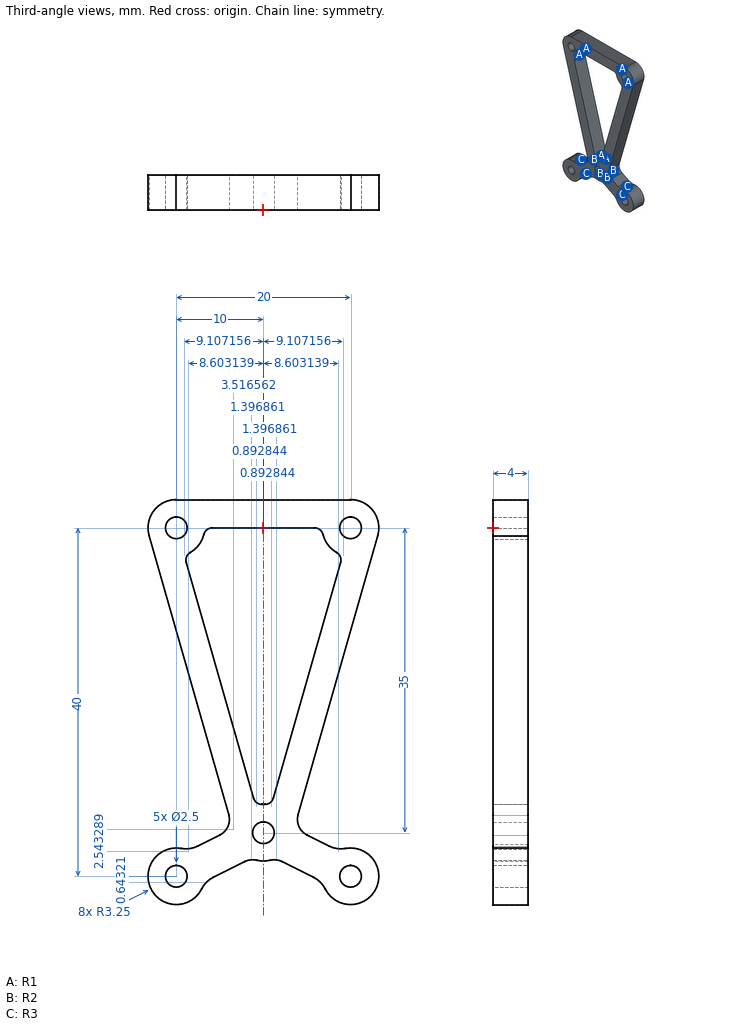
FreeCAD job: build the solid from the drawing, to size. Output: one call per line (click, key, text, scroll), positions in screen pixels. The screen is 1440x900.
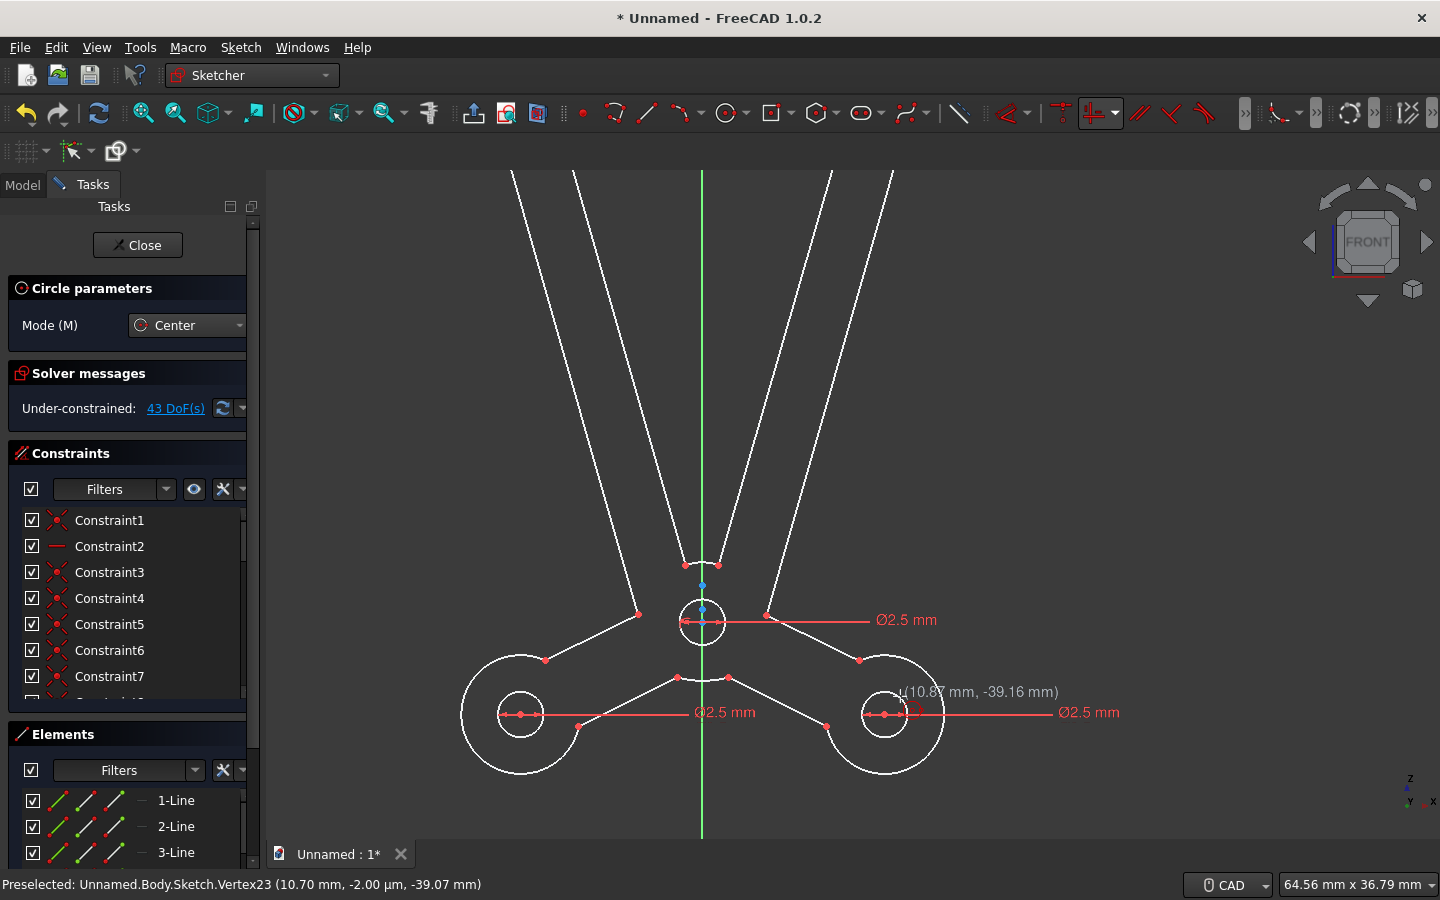
scroll(884, 714, down, 3)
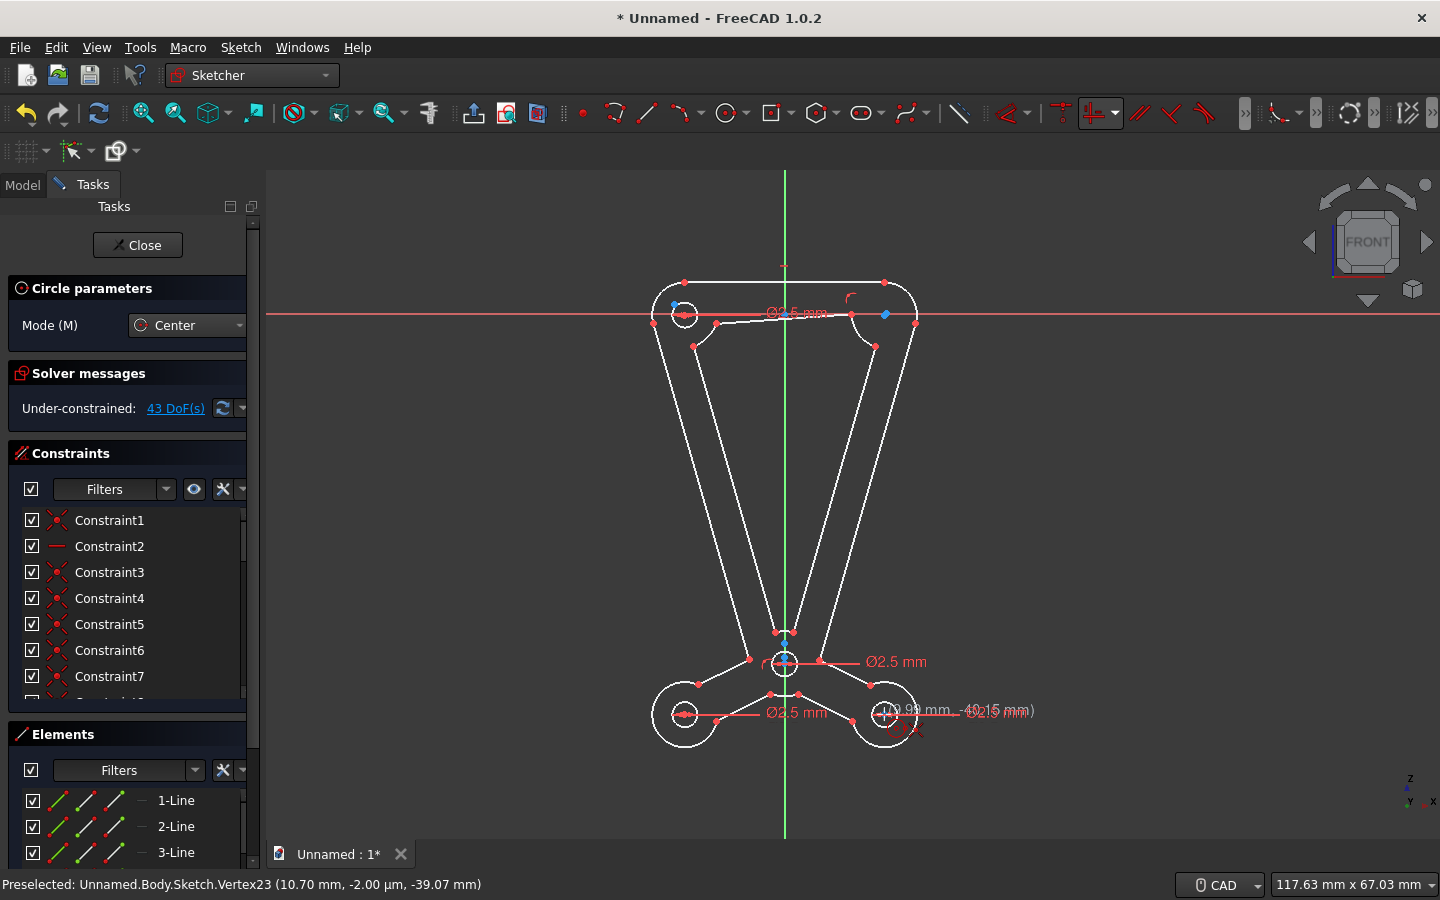
scroll(884, 314, up, 3)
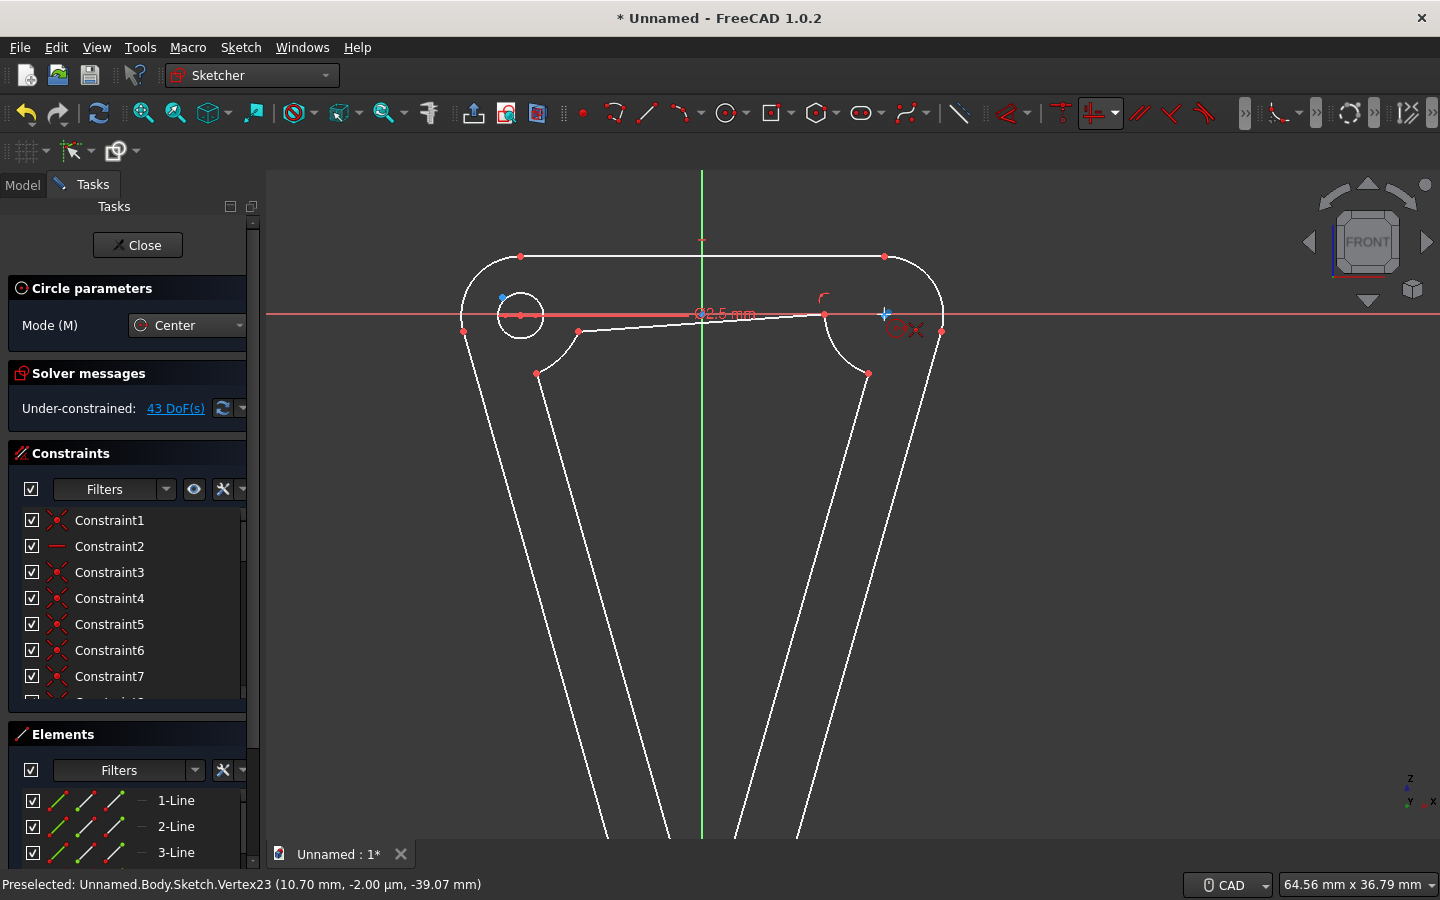
click(884, 314)
move(900, 298)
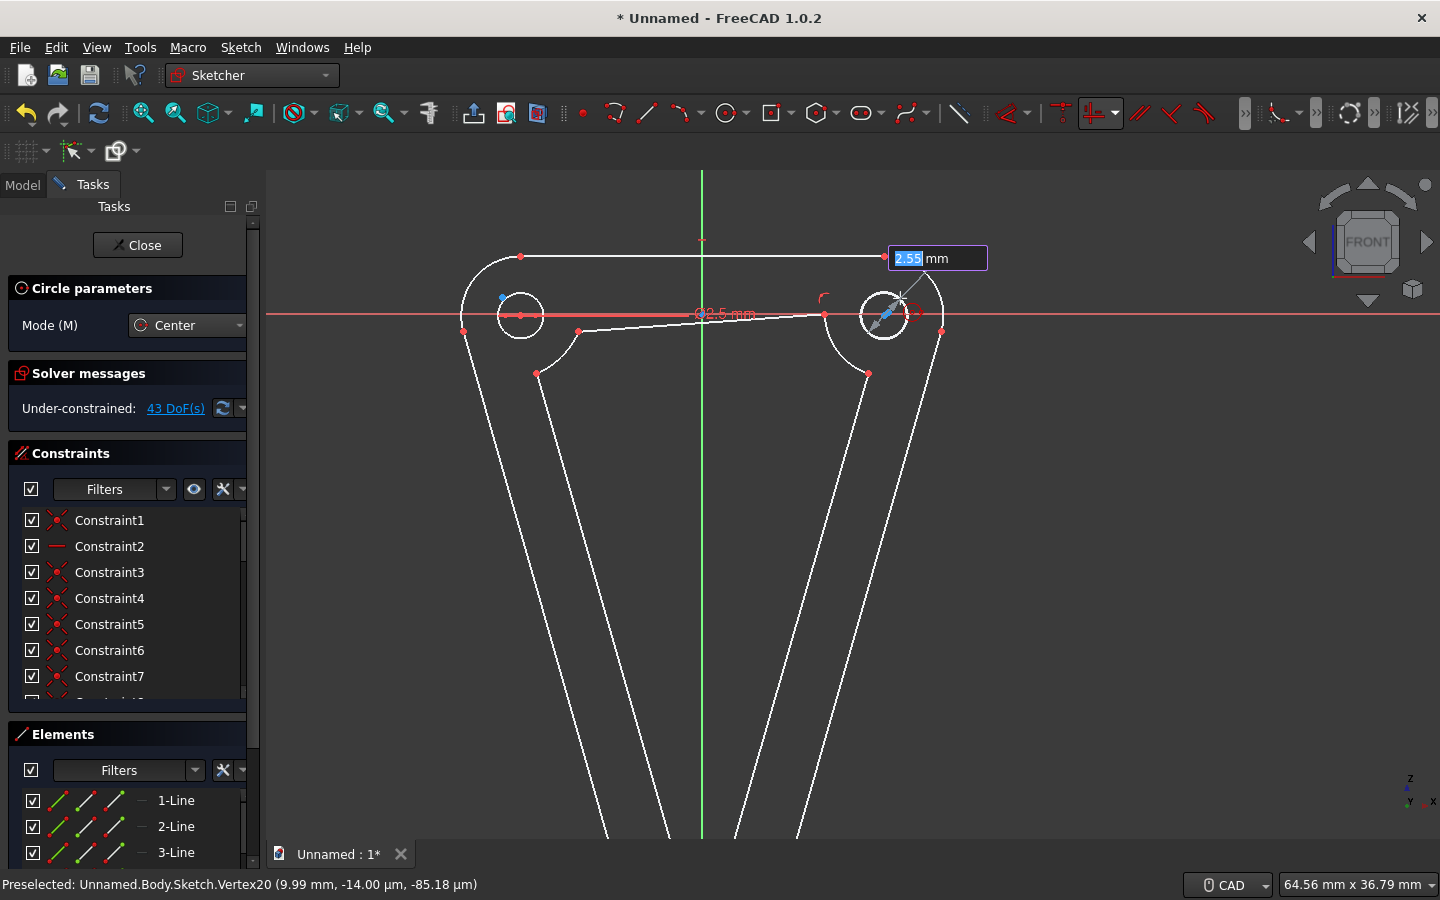
text(2.5)
key(Return)
key(Escape)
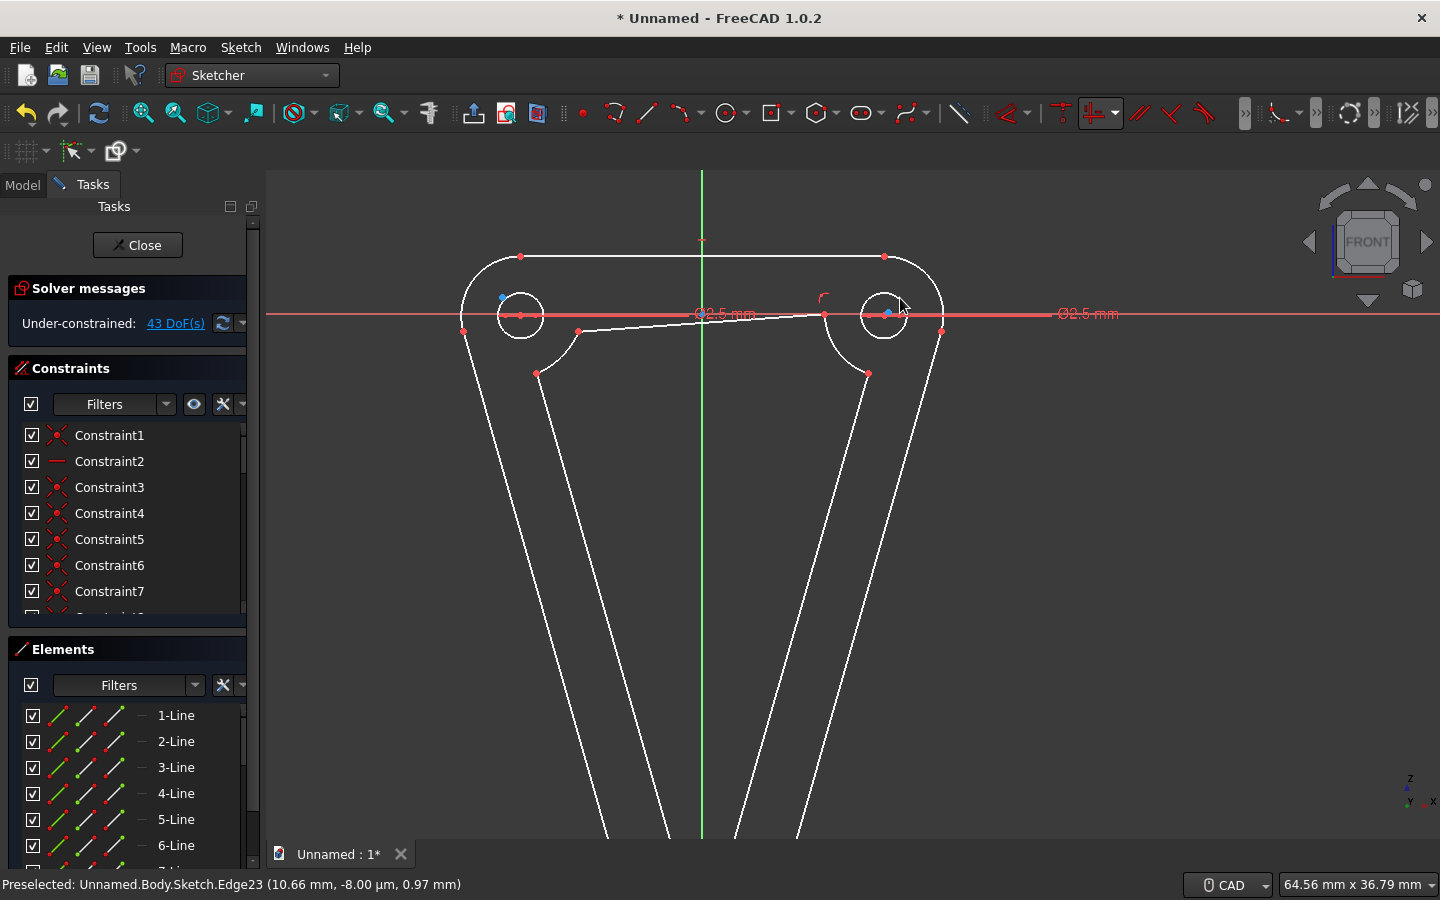
click(586, 760)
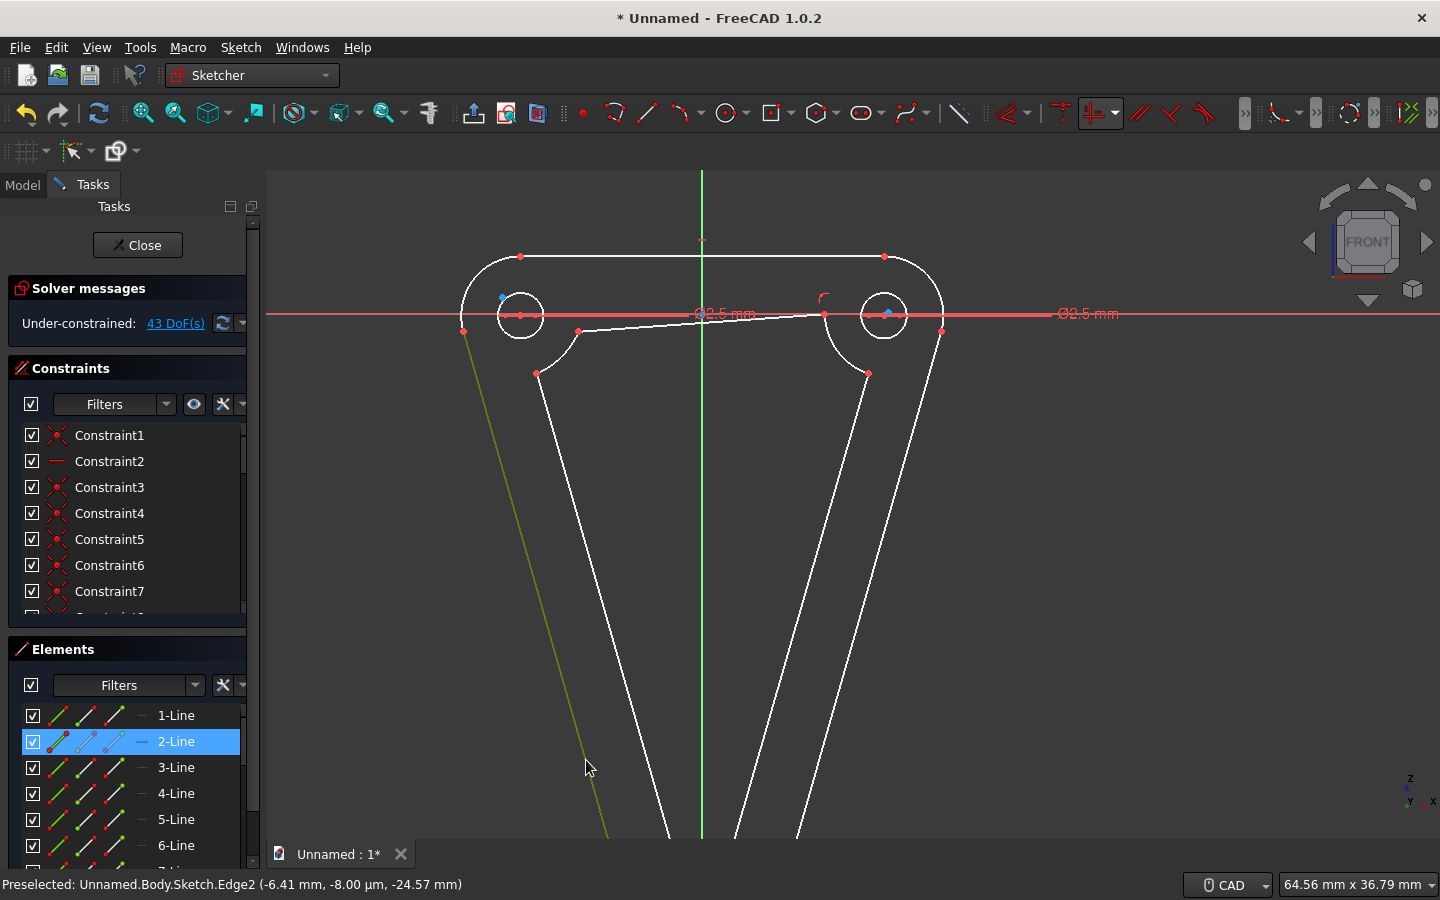
click(489, 265)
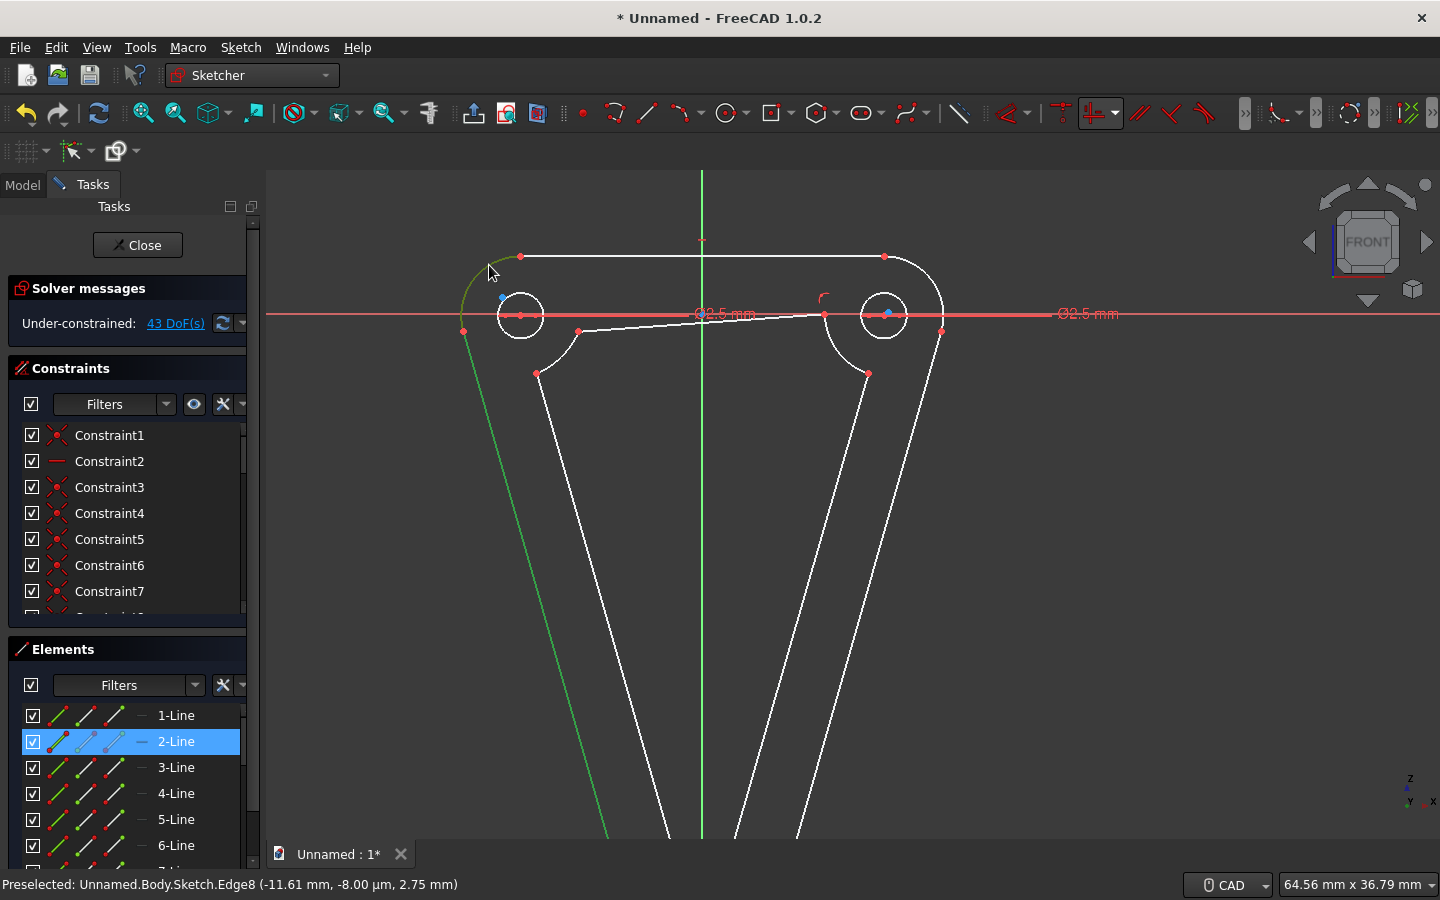
click(1204, 114)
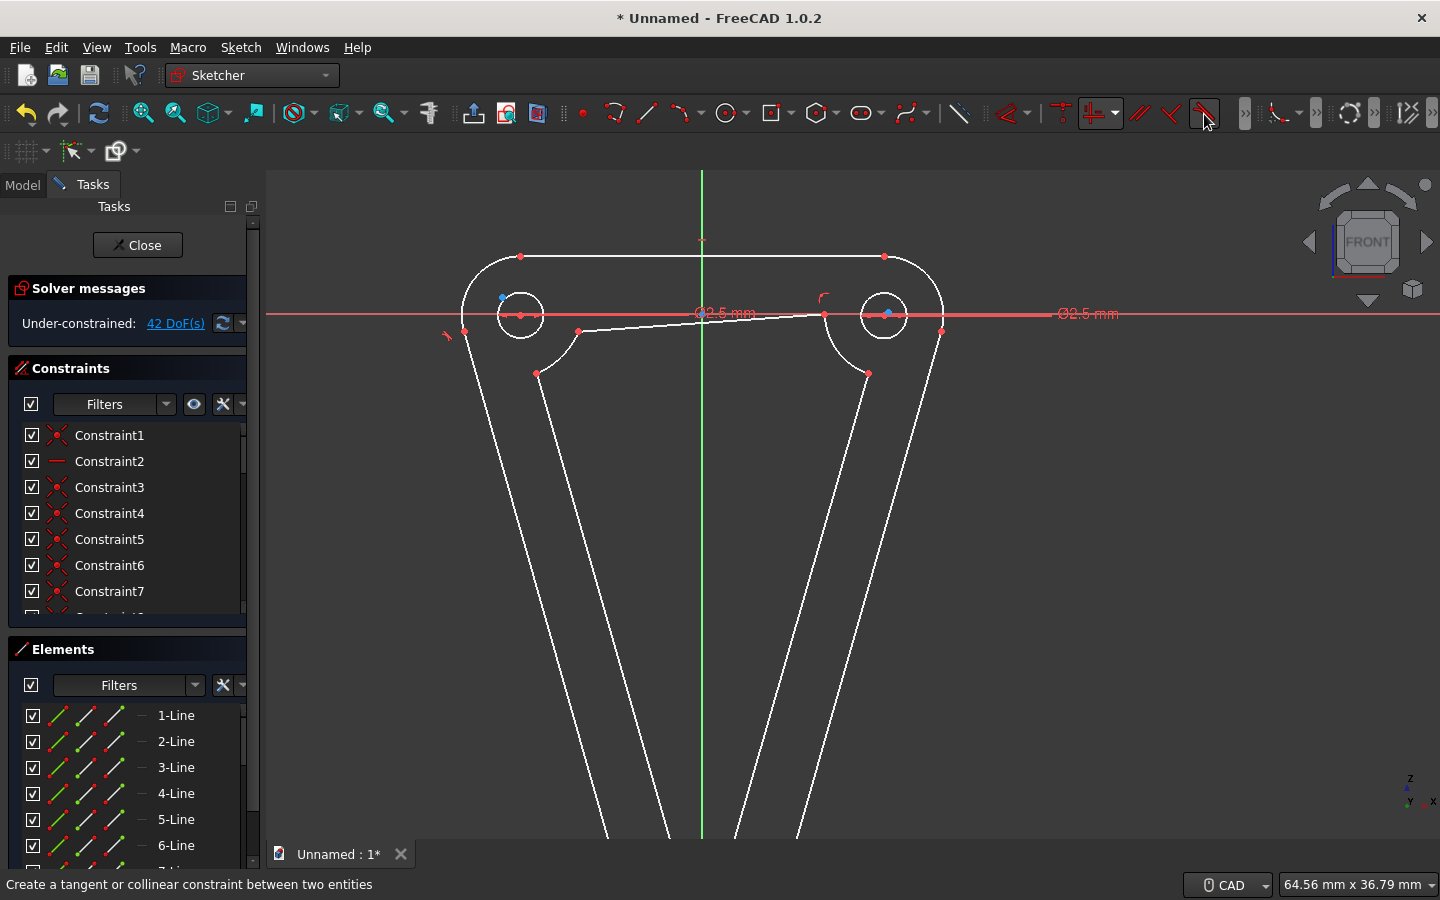
click(630, 256)